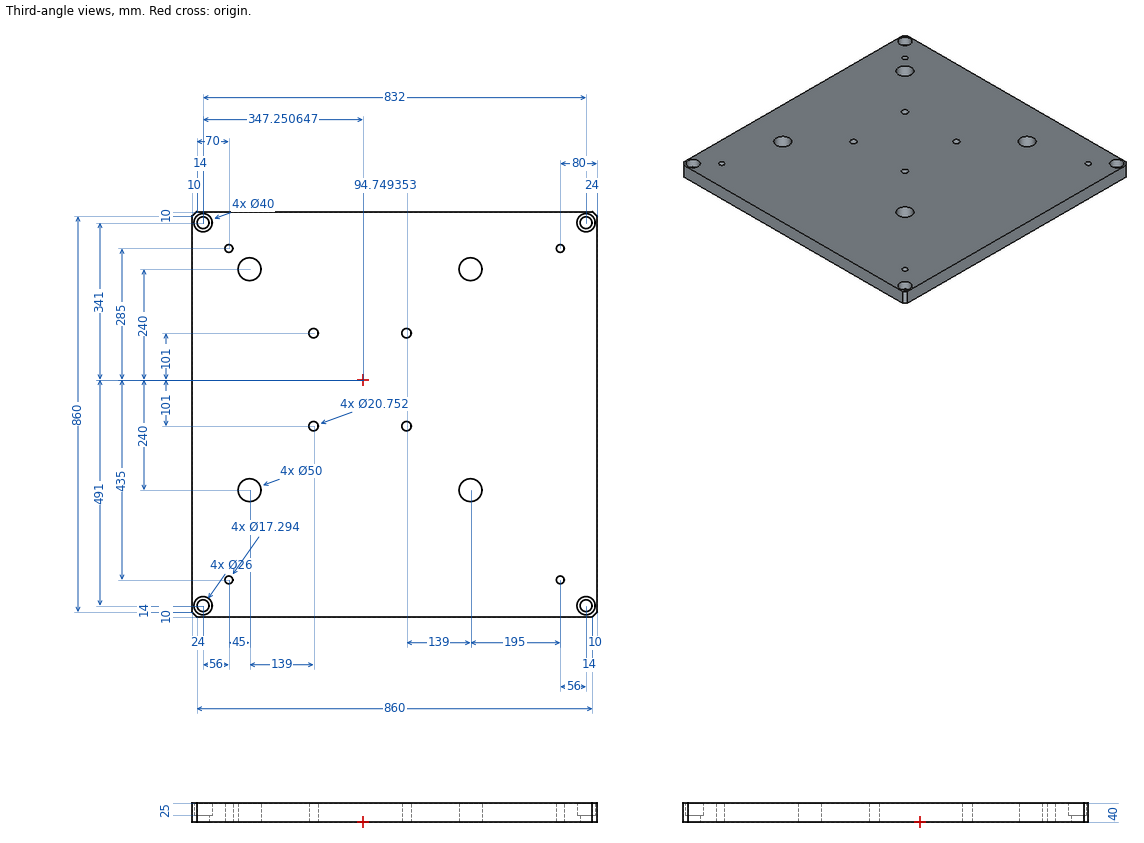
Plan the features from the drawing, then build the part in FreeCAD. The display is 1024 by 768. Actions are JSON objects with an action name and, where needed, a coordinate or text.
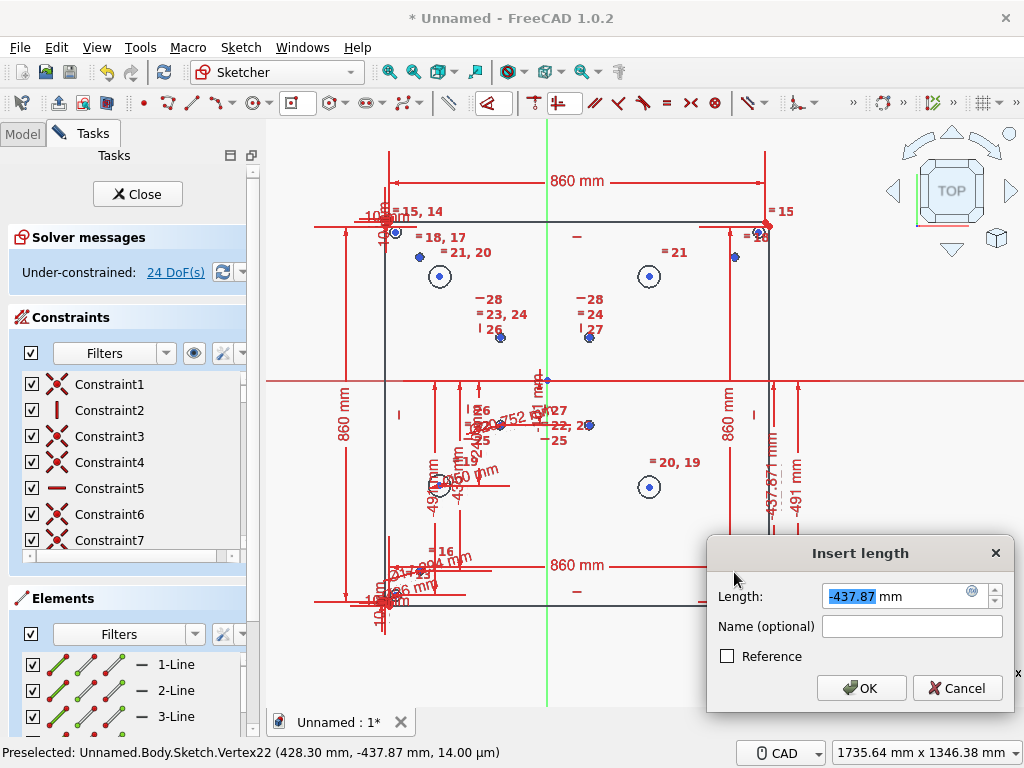
{"action": "type", "text": "-435"}
{"action": "key", "text": "Return"}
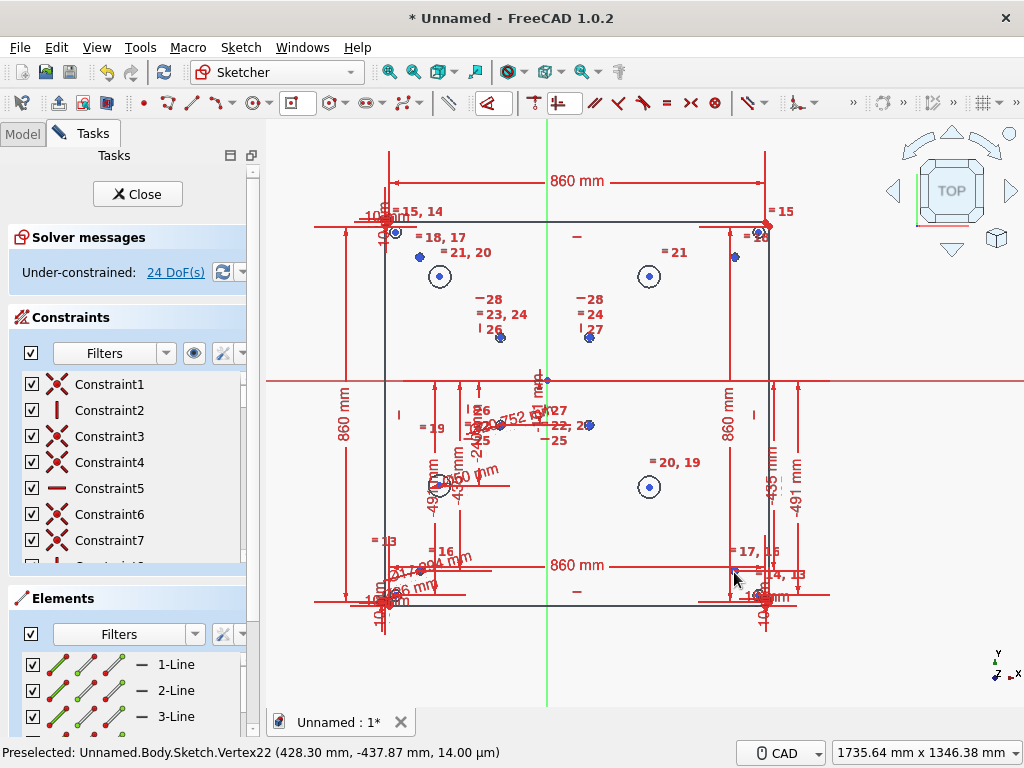
{"action": "left_click", "coordinate": [649, 487]}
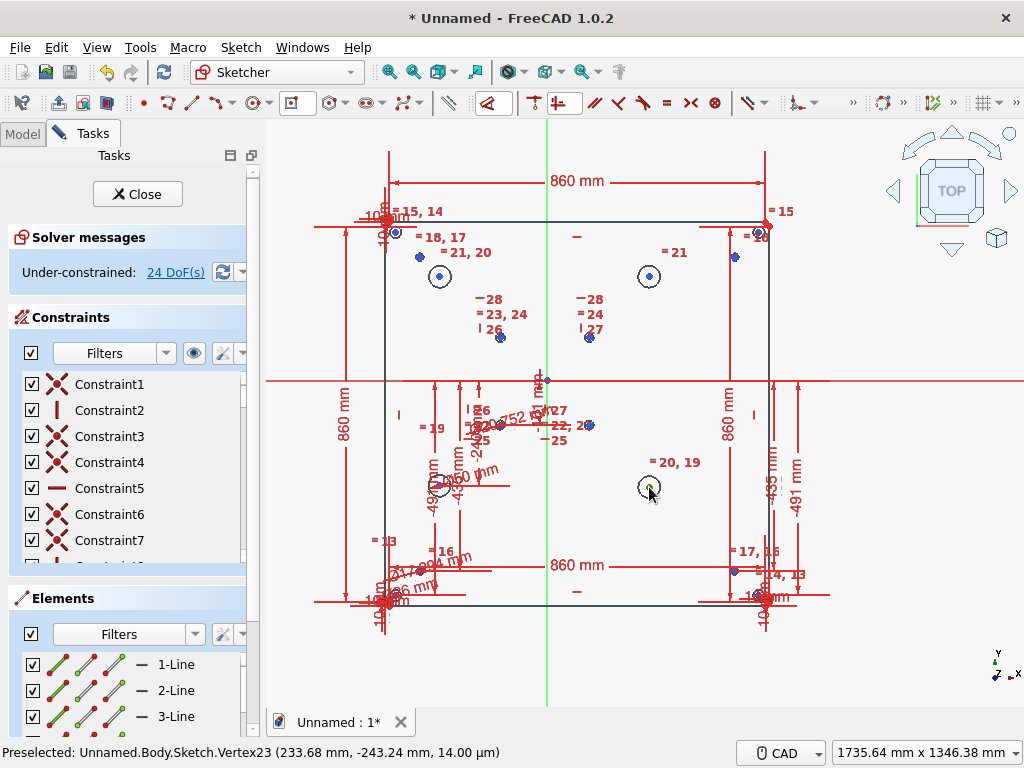
{"action": "key", "text": "i"}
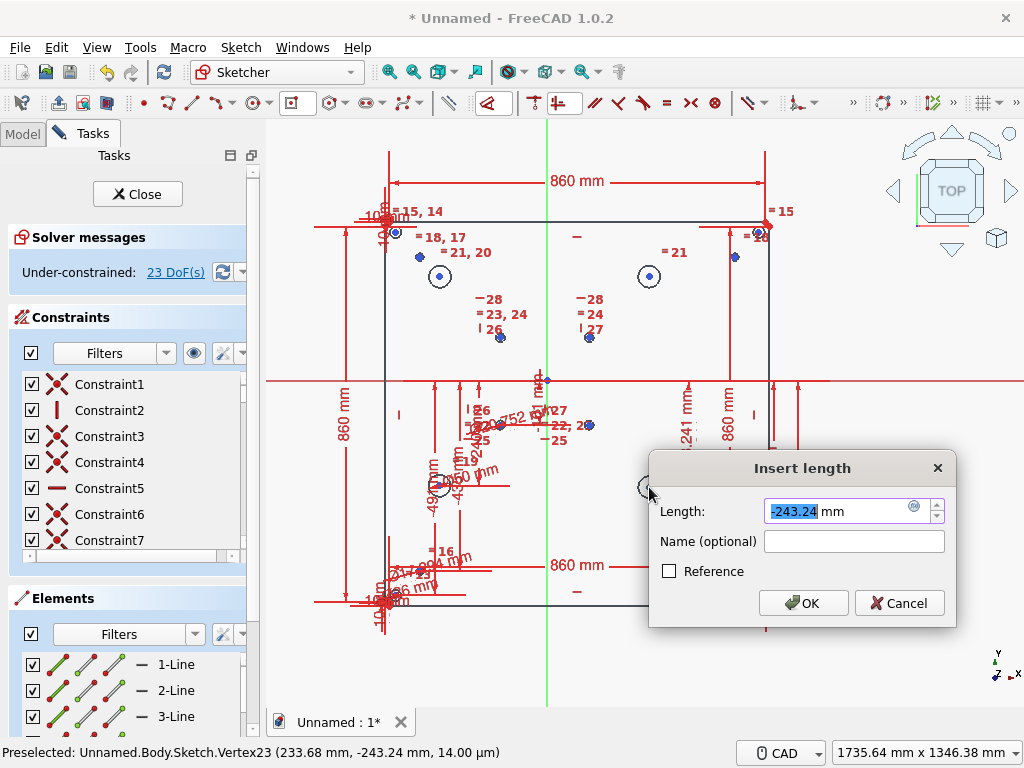
{"action": "type", "text": "-240"}
{"action": "key", "text": "Return"}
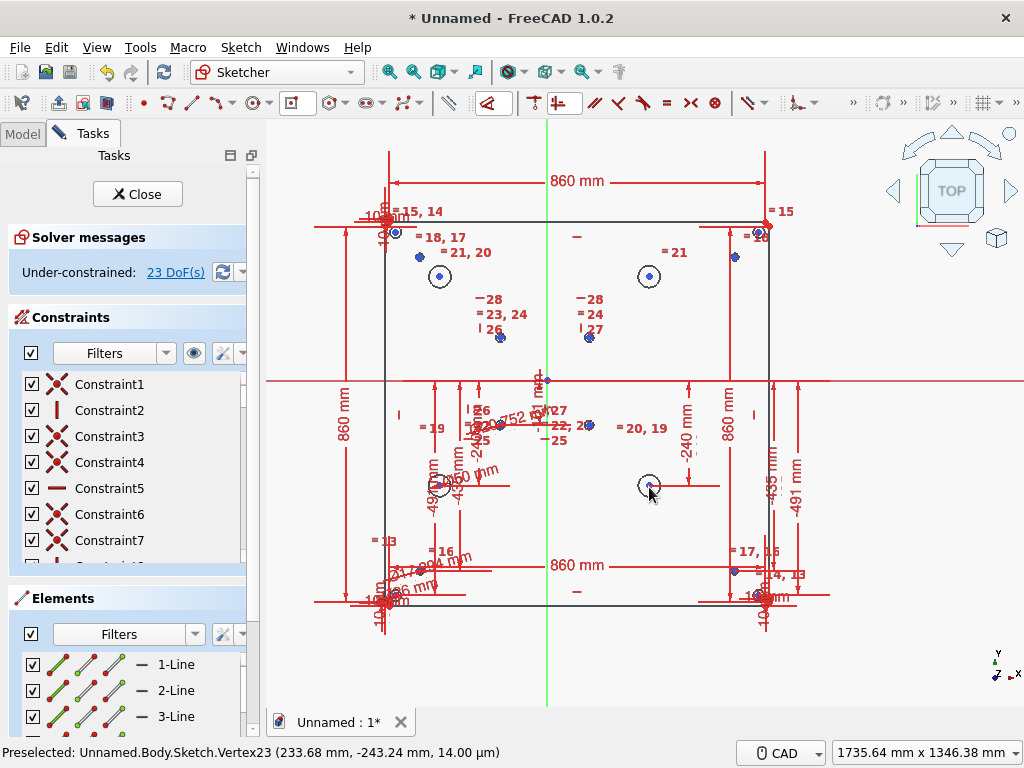
{"action": "left_click", "coordinate": [500, 338]}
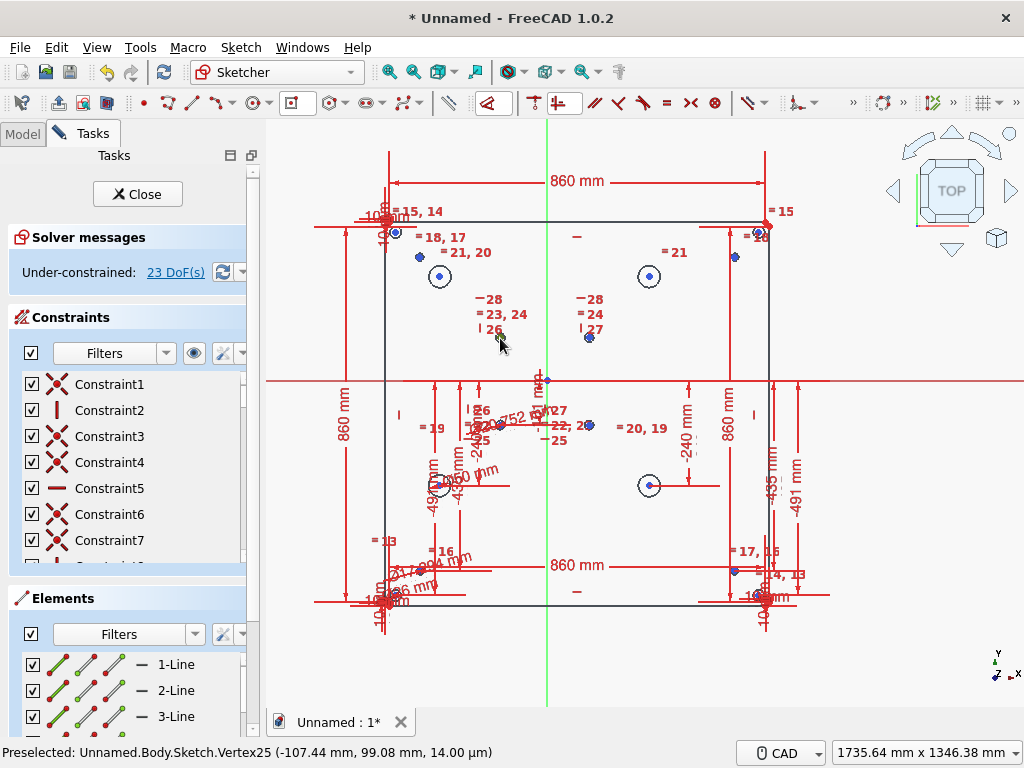
{"action": "left_click", "coordinate": [506, 104]}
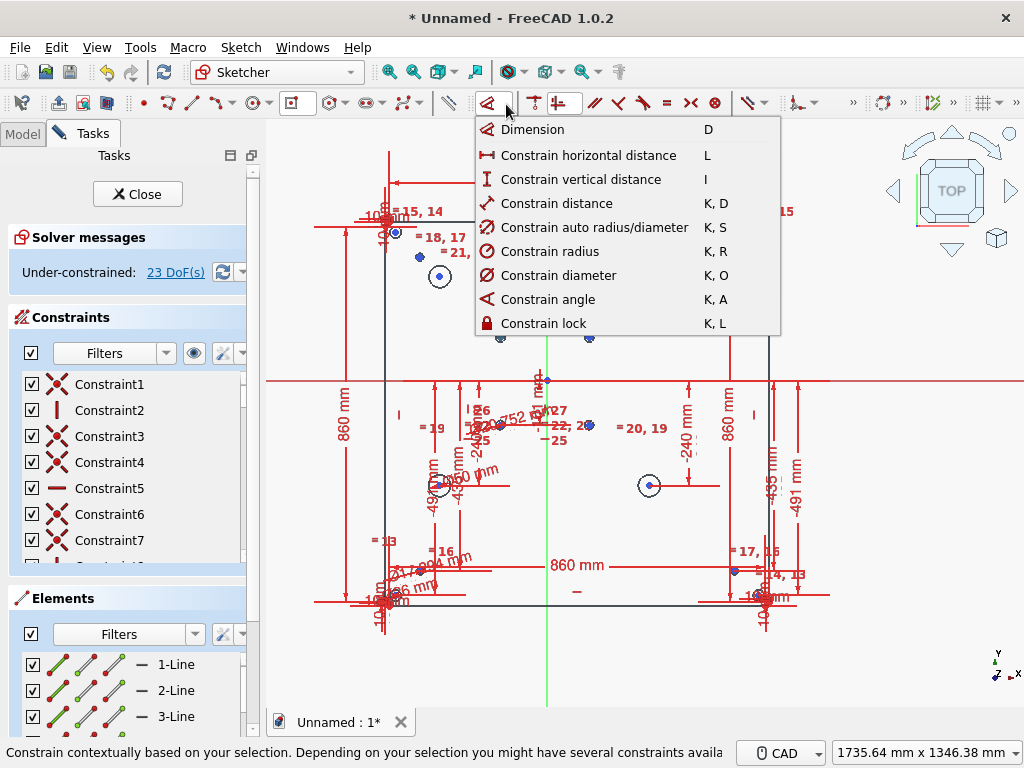
{"action": "left_click", "coordinate": [628, 179]}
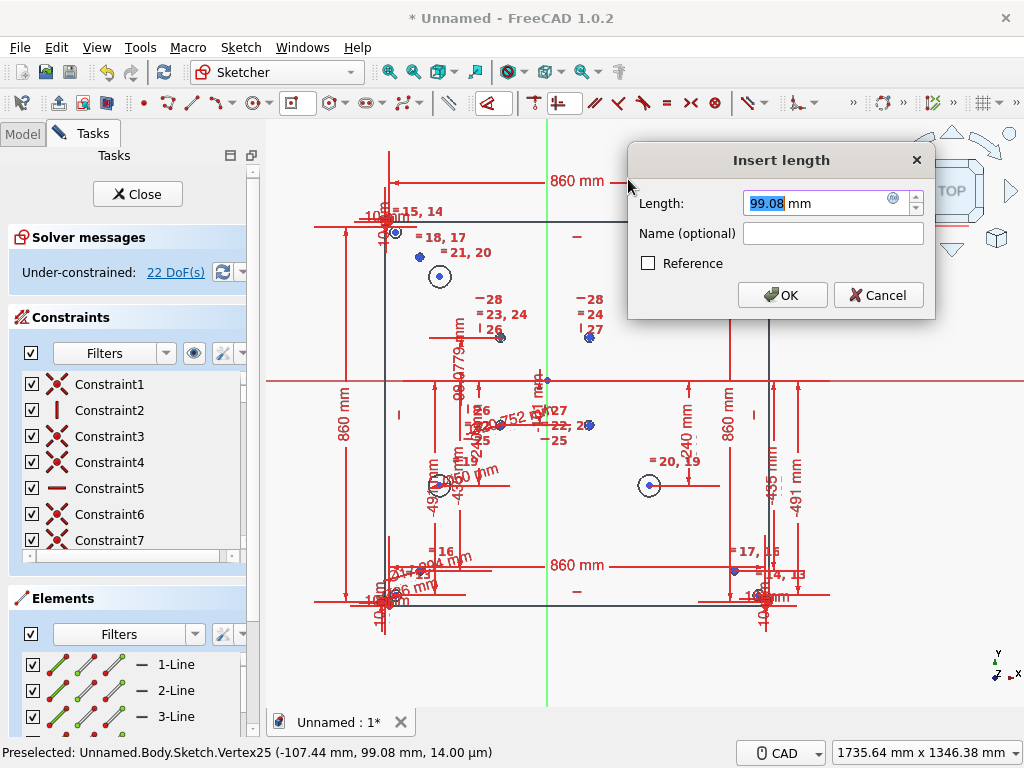
{"action": "type", "text": "101"}
{"action": "key", "text": "Return"}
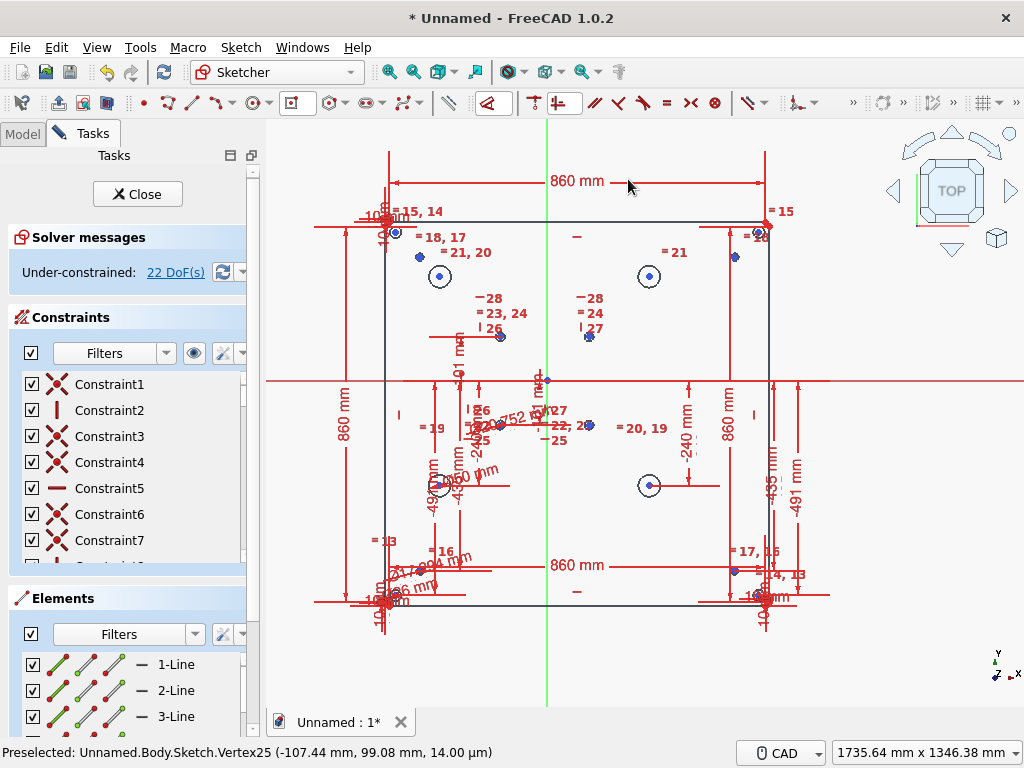
{"action": "left_click", "coordinate": [440, 277]}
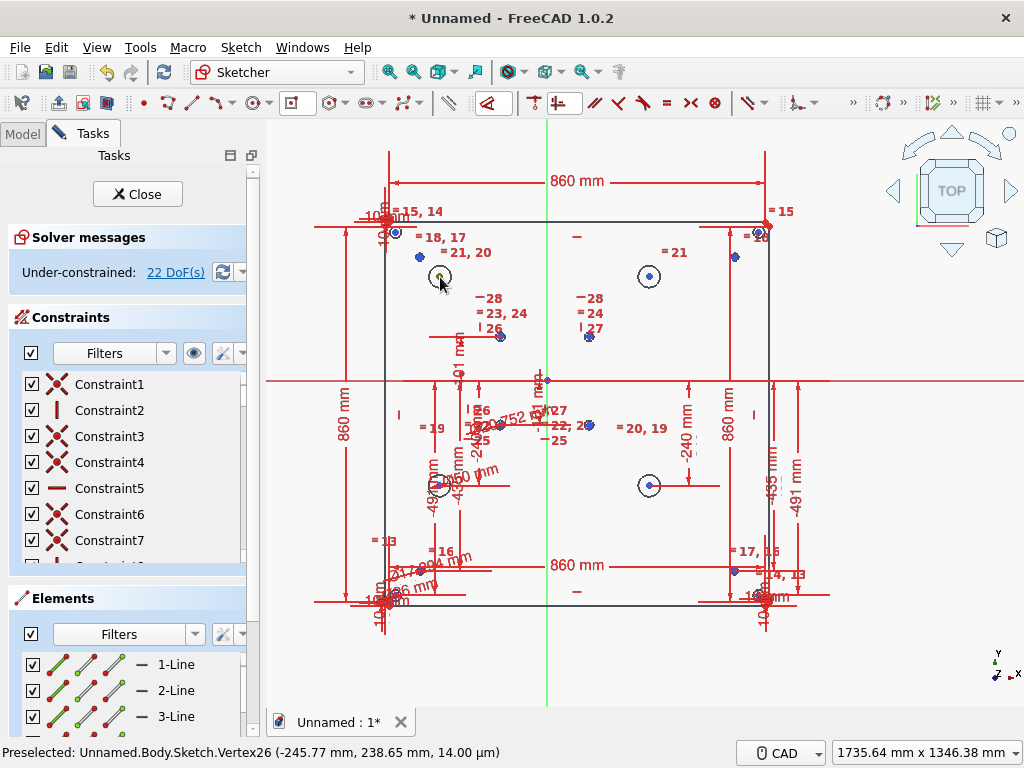
{"action": "key", "text": "i"}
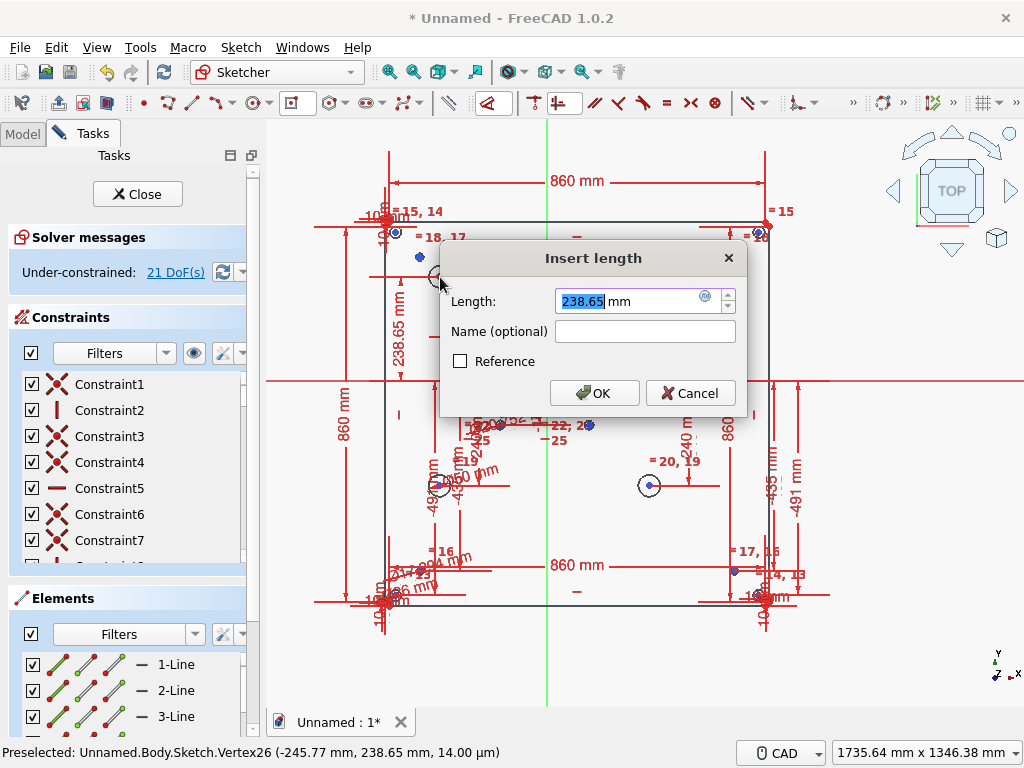
{"action": "type", "text": "240"}
{"action": "key", "text": "Return"}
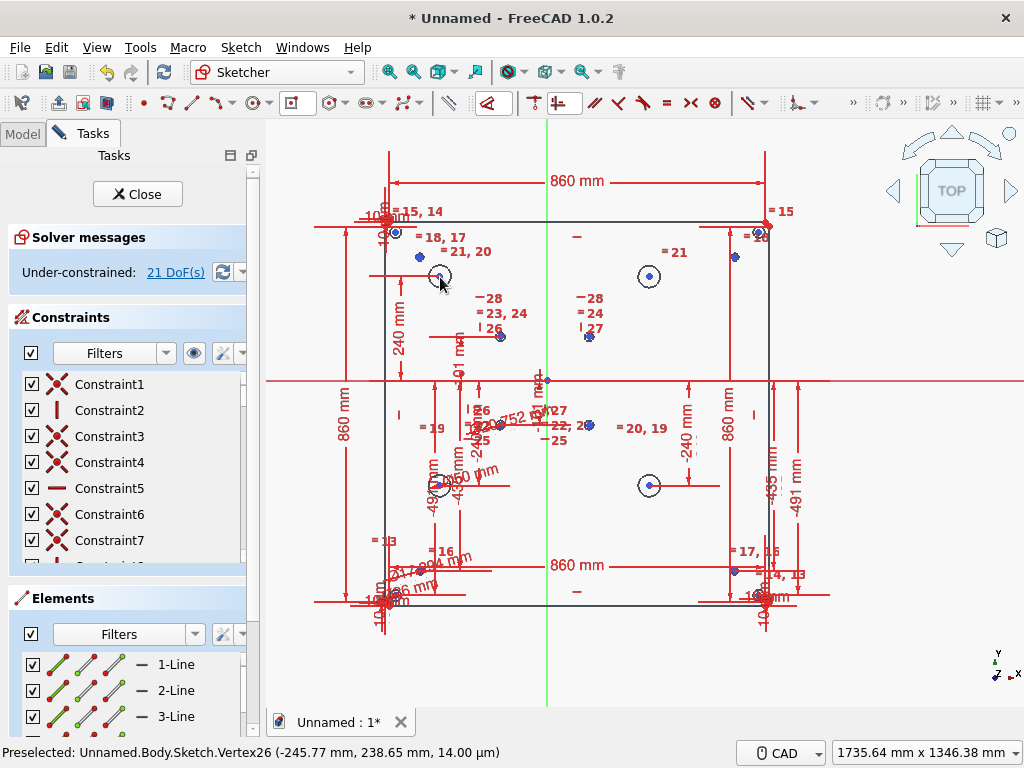
{"action": "left_click", "coordinate": [420, 257]}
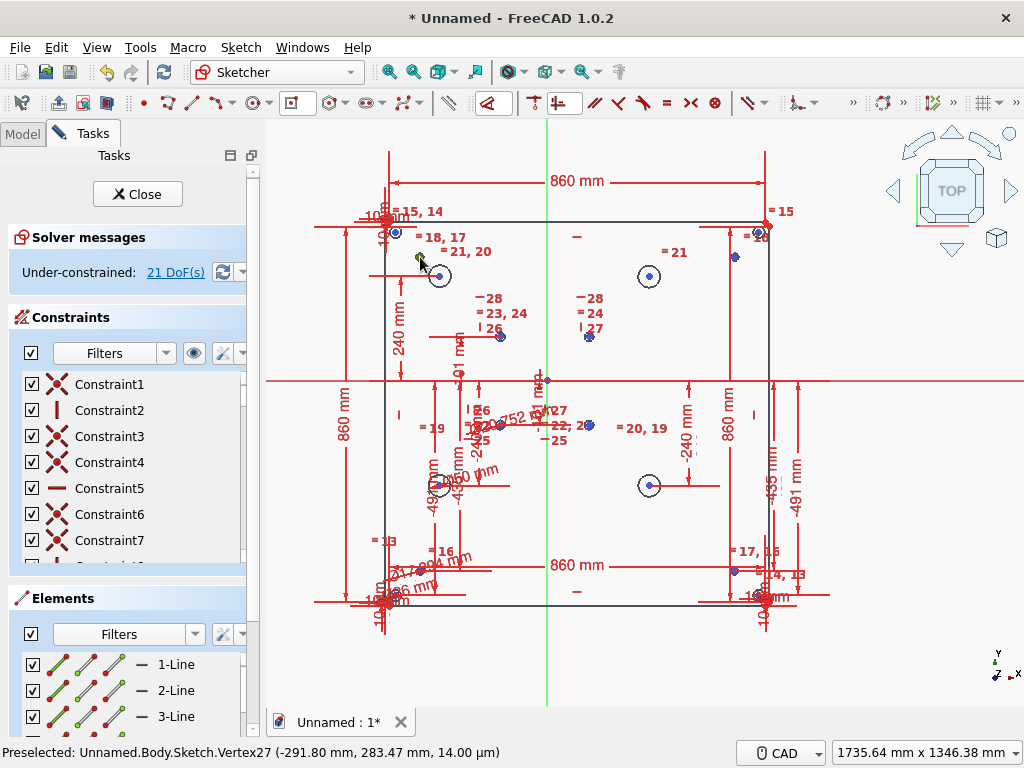
{"action": "key", "text": "i"}